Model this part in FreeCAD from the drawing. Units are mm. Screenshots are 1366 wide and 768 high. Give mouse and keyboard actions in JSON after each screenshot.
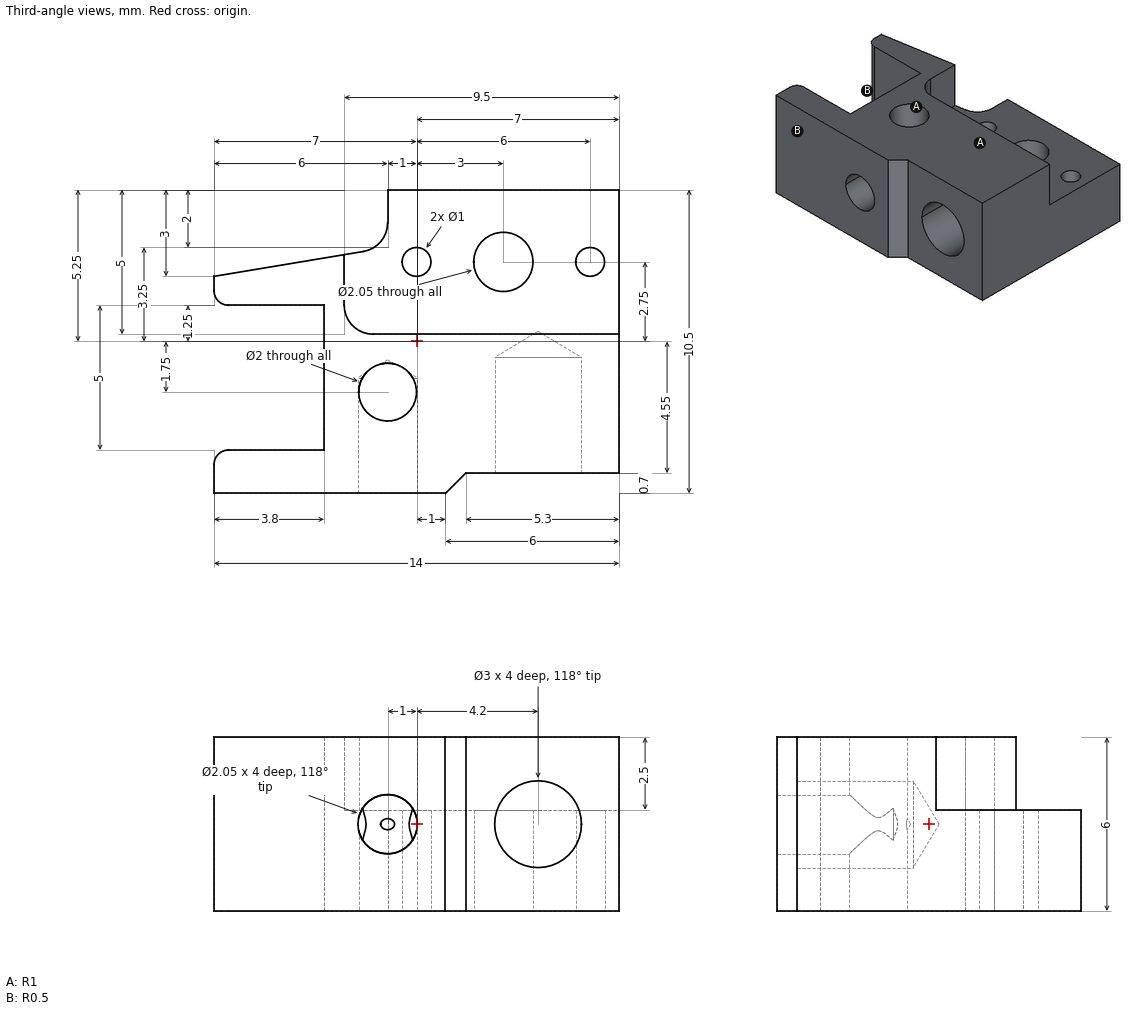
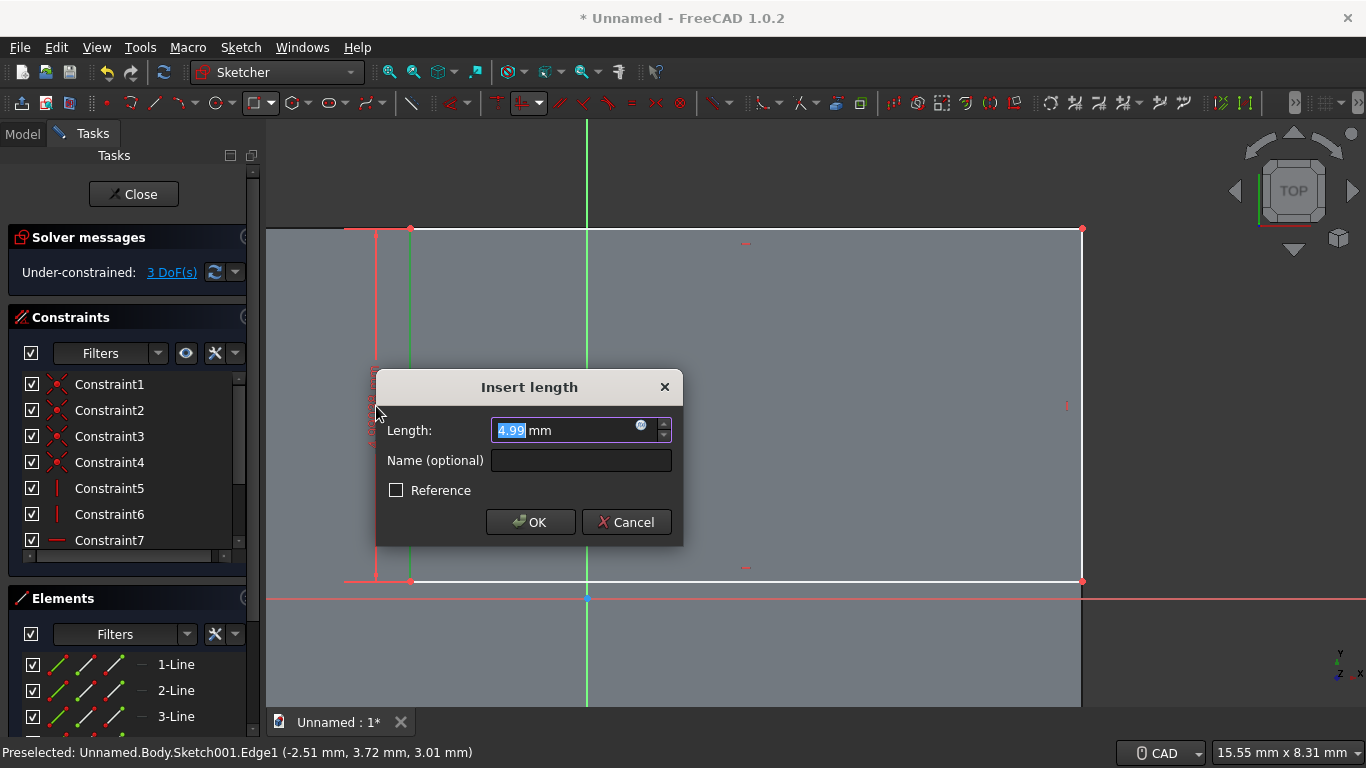
{"action": "type", "text": "5"}
{"action": "key", "text": "Return"}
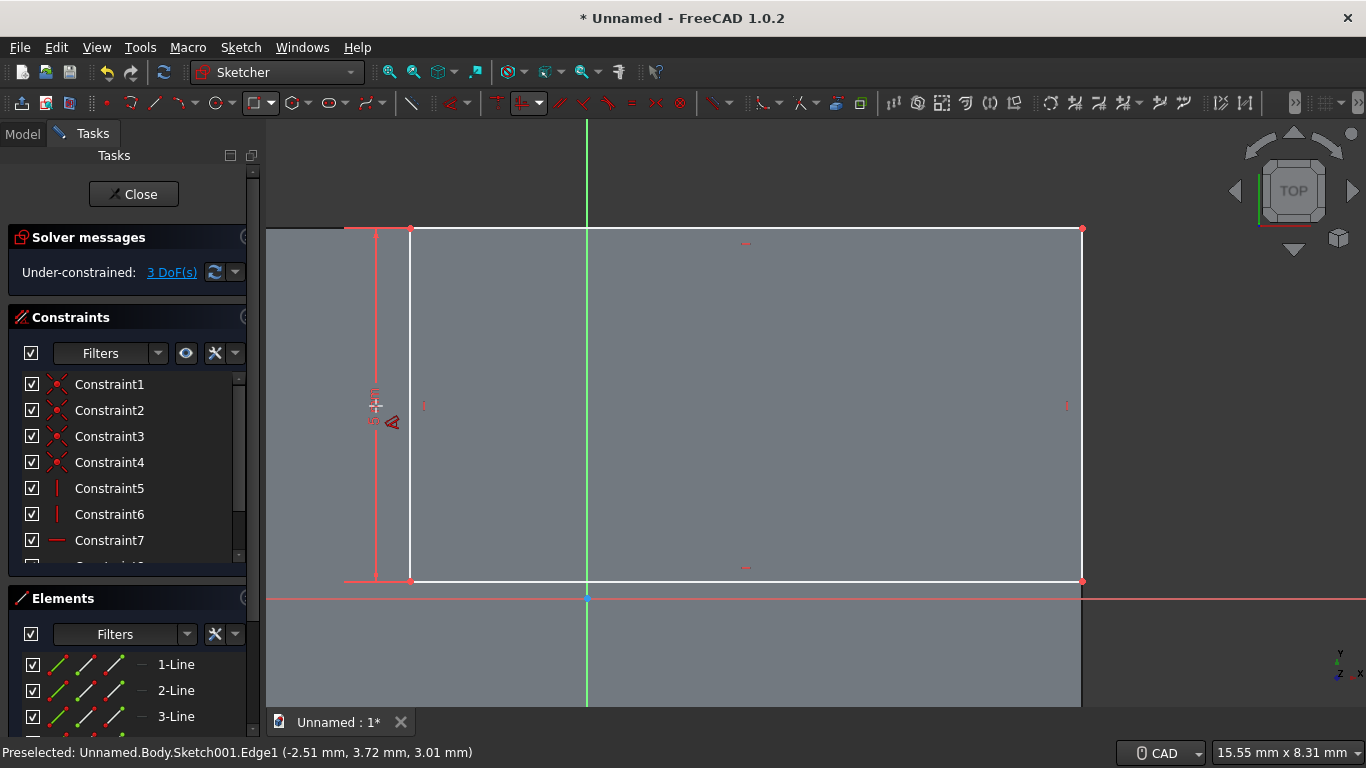
{"action": "left_click", "coordinate": [1082, 582]}
{"action": "left_click", "coordinate": [835, 633]}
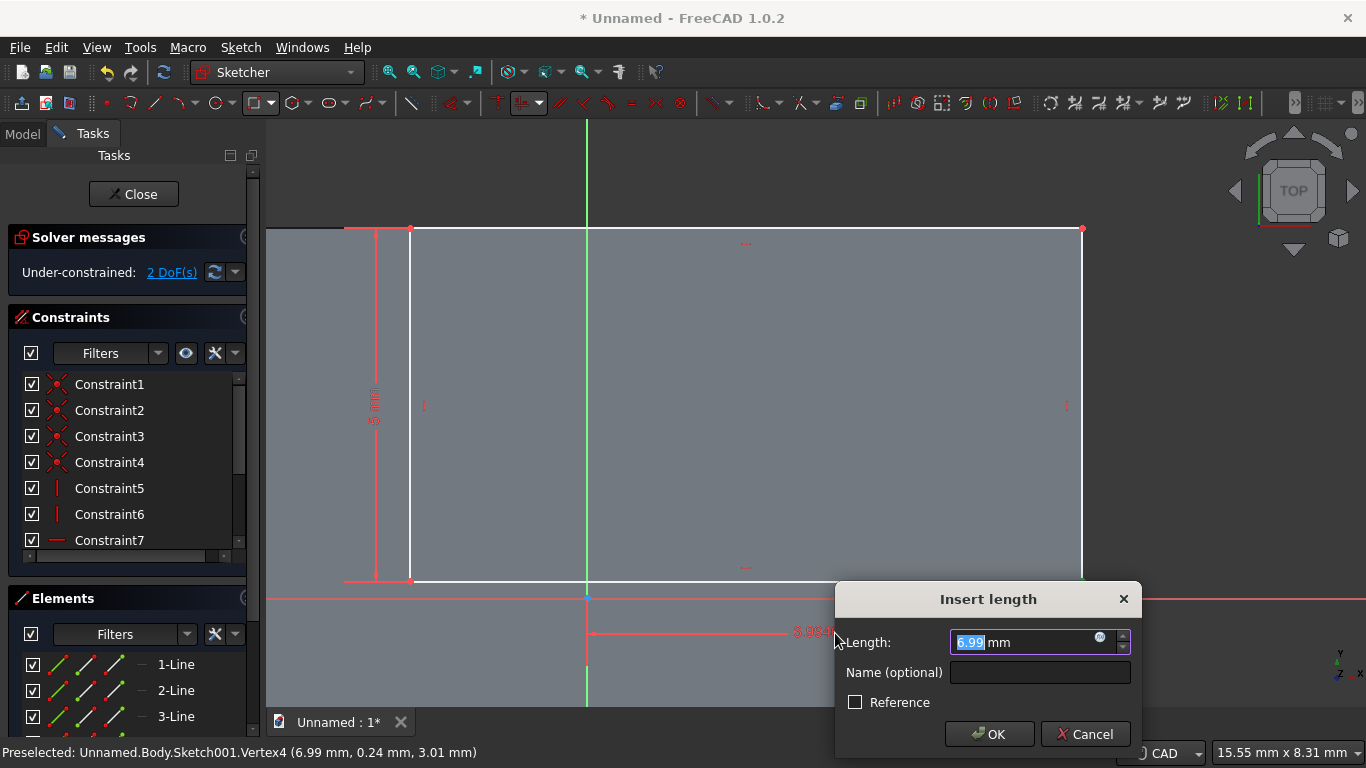
{"action": "type", "text": "7"}
{"action": "key", "text": "Return"}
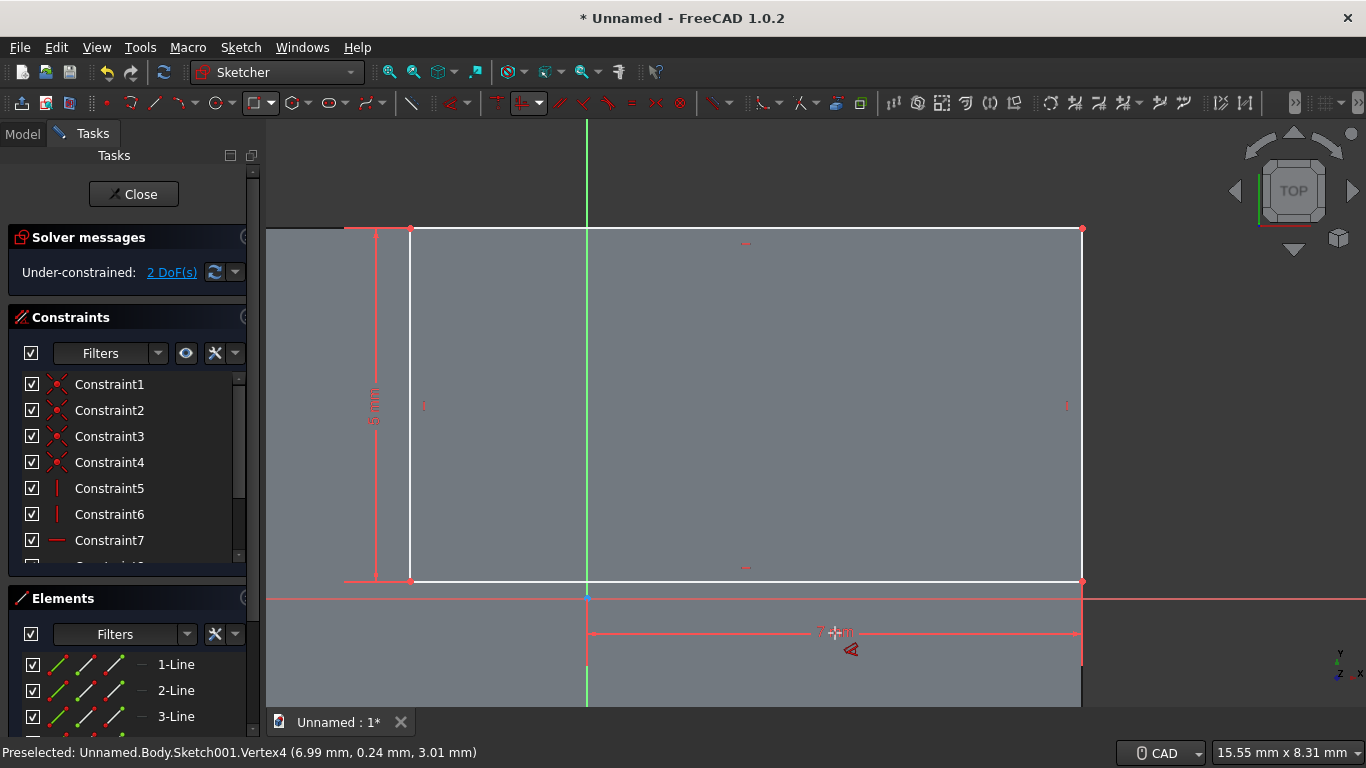
{"action": "left_click", "coordinate": [612, 582]}
{"action": "left_click", "coordinate": [746, 616]}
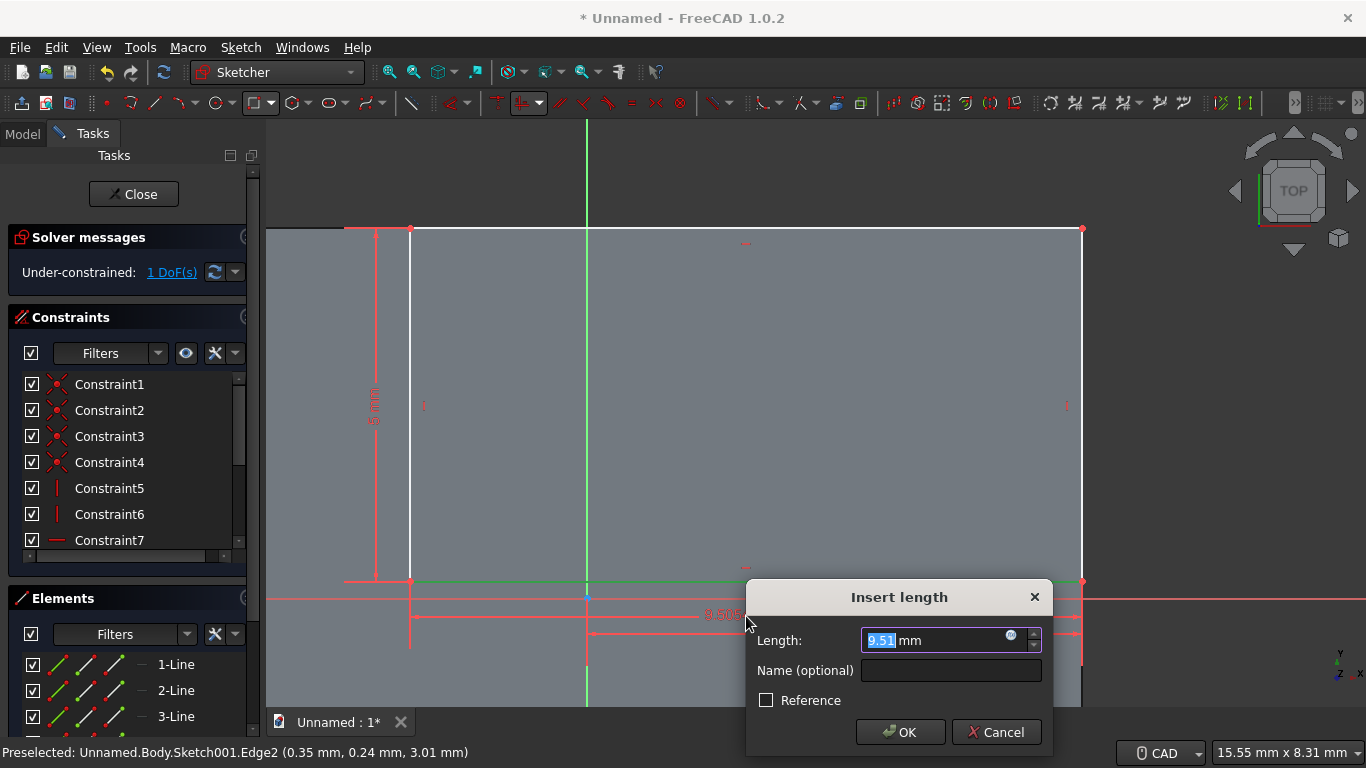
{"action": "type", "text": "9.5"}
{"action": "key", "text": "Return"}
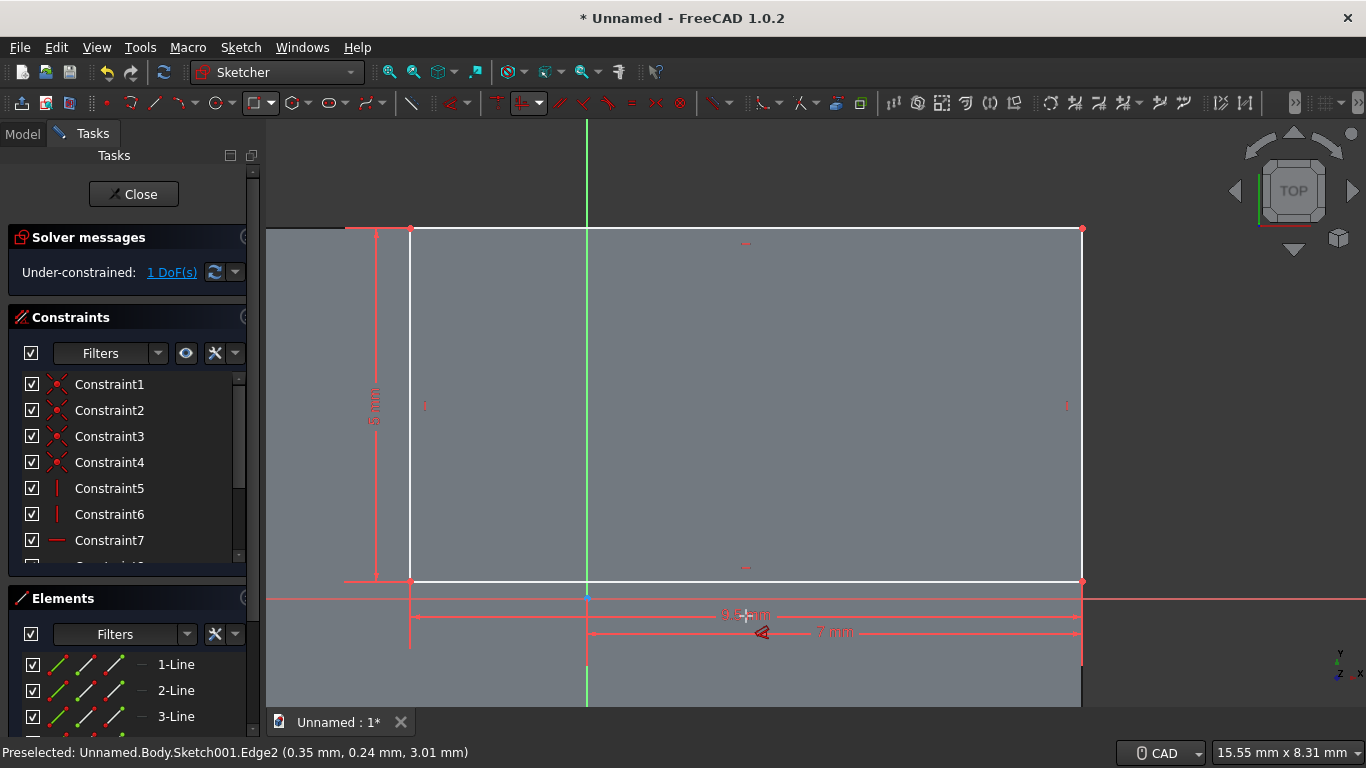
{"action": "left_click", "coordinate": [410, 228]}
{"action": "left_click", "coordinate": [376, 328]}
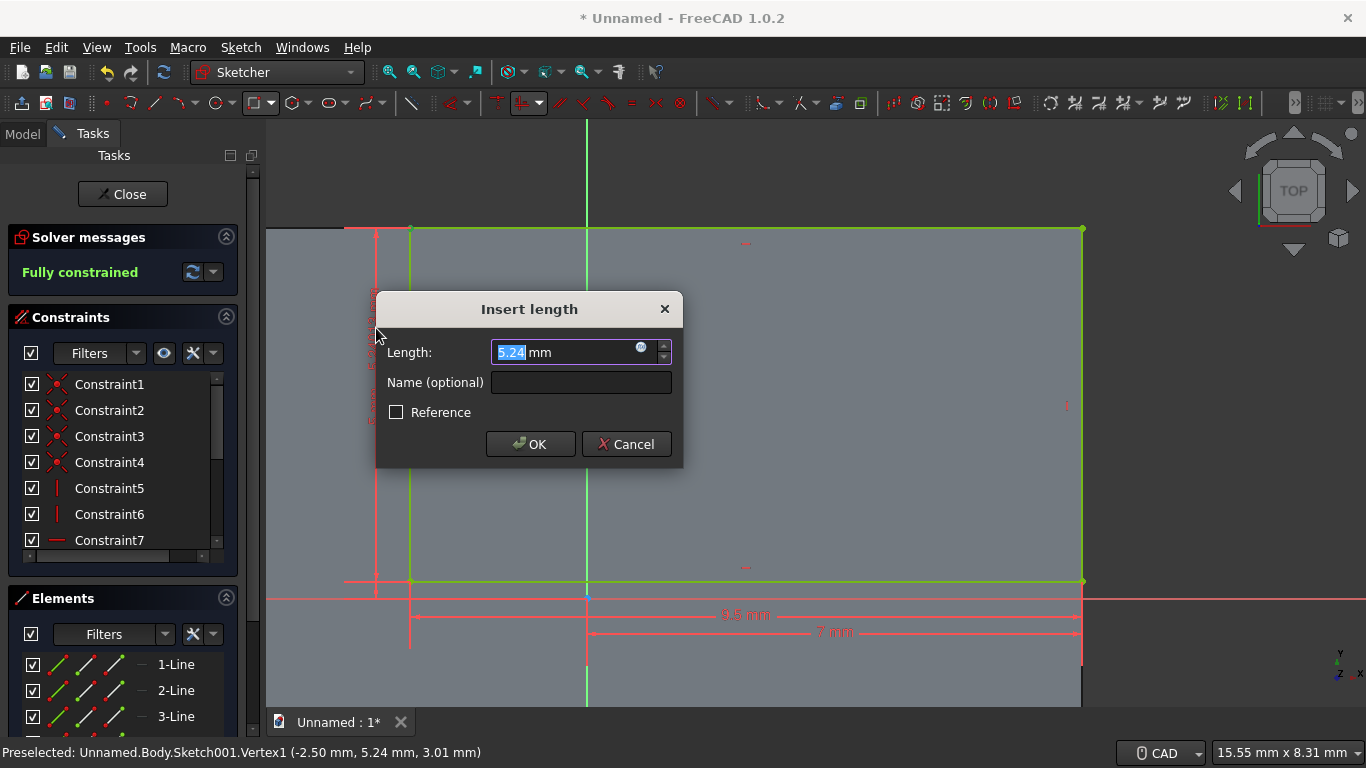
{"action": "type", "text": "5.25"}
{"action": "key", "text": "Return"}
{"action": "key", "text": "Escape"}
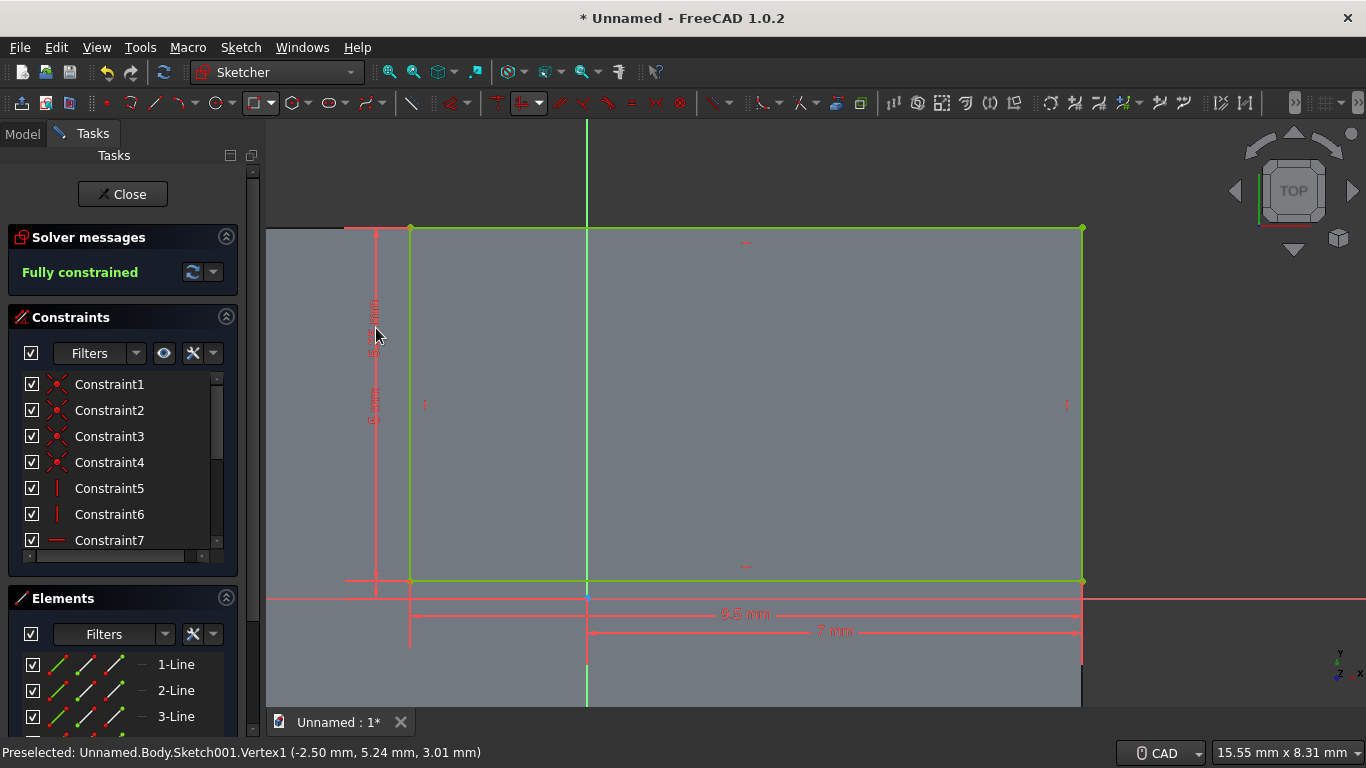
{"action": "left_click", "coordinate": [123, 194]}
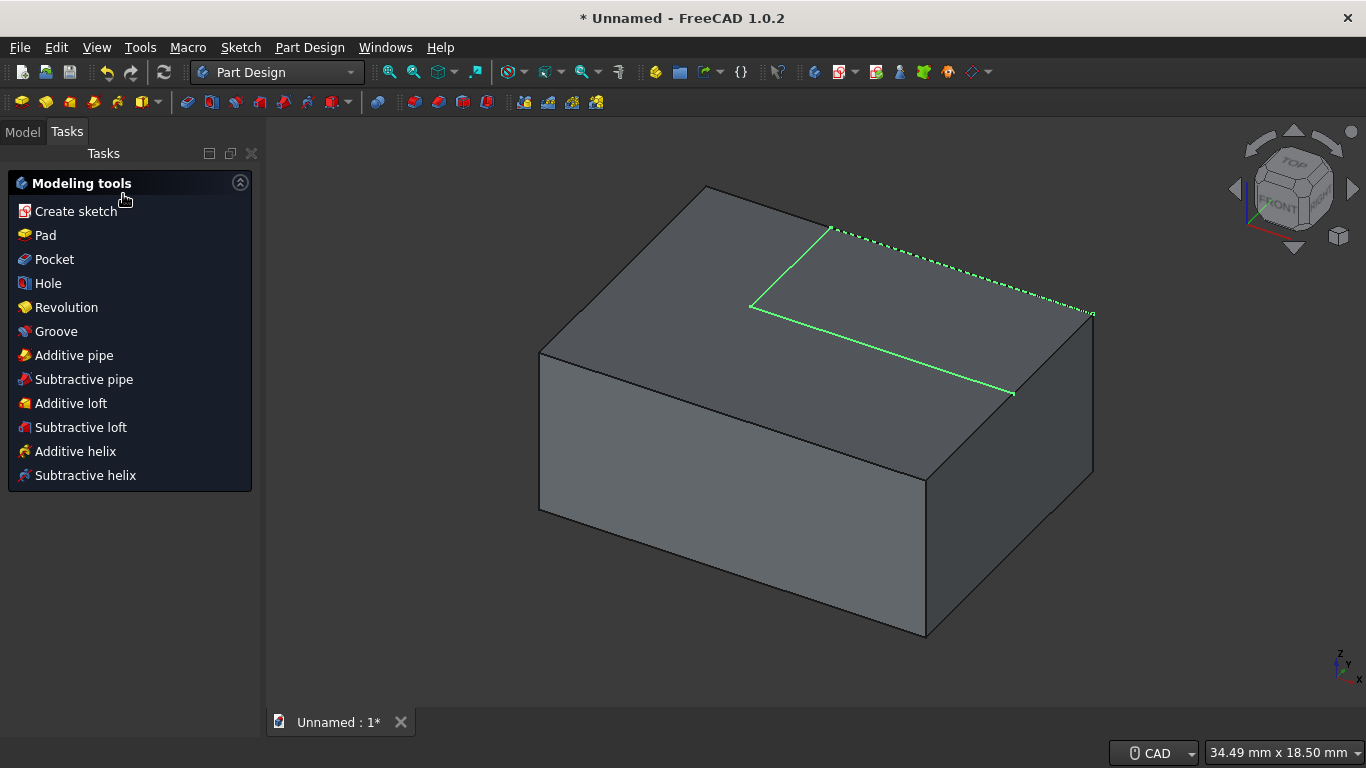
{"action": "left_click", "coordinate": [188, 102]}